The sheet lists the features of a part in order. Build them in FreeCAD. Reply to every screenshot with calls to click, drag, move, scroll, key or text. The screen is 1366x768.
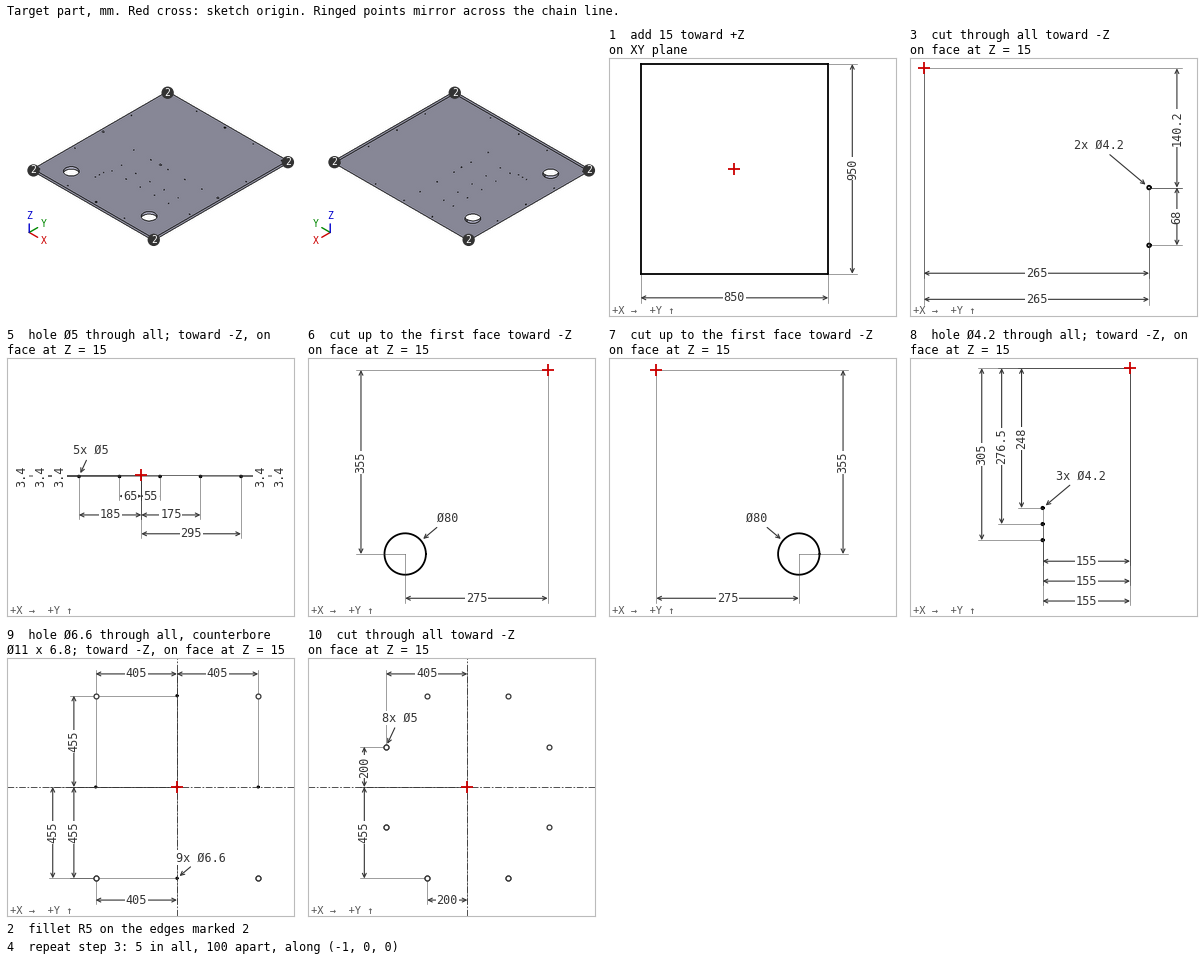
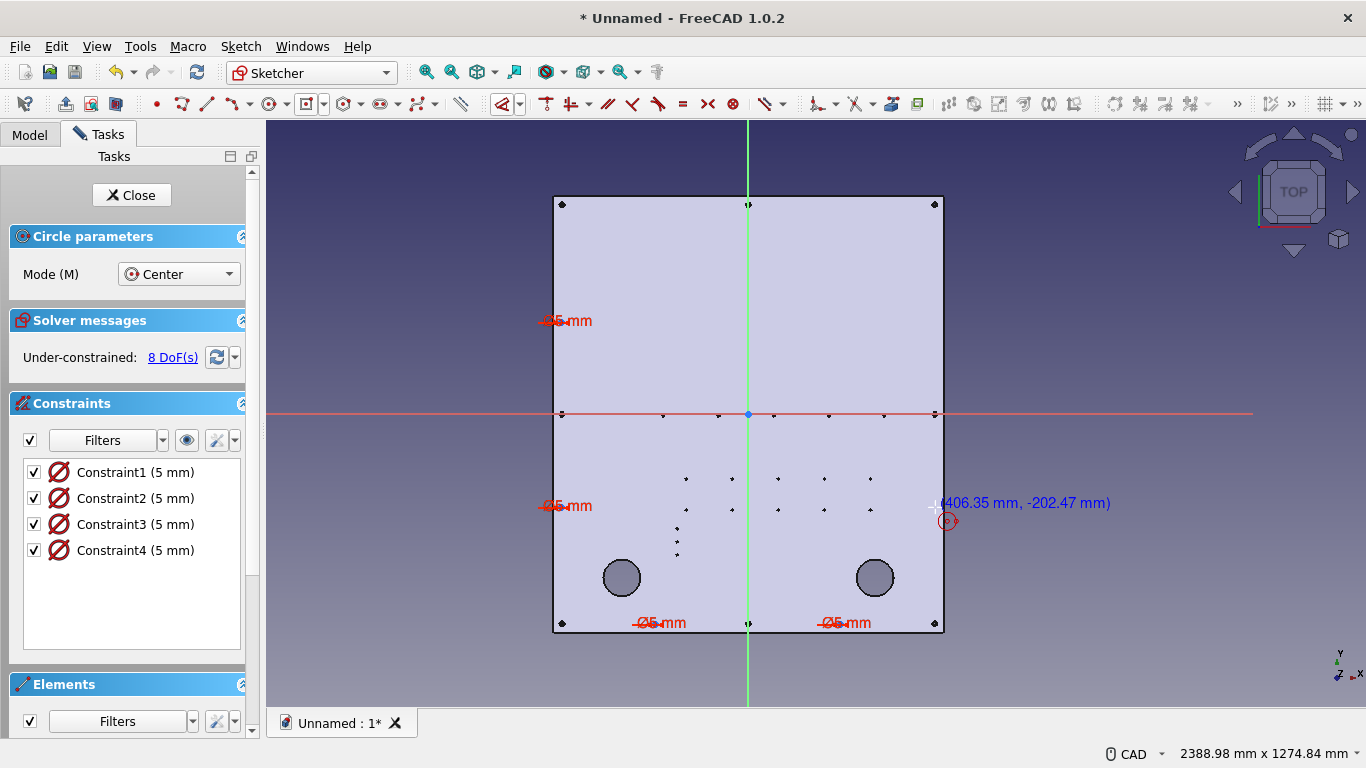
click(935, 507)
move(936, 506)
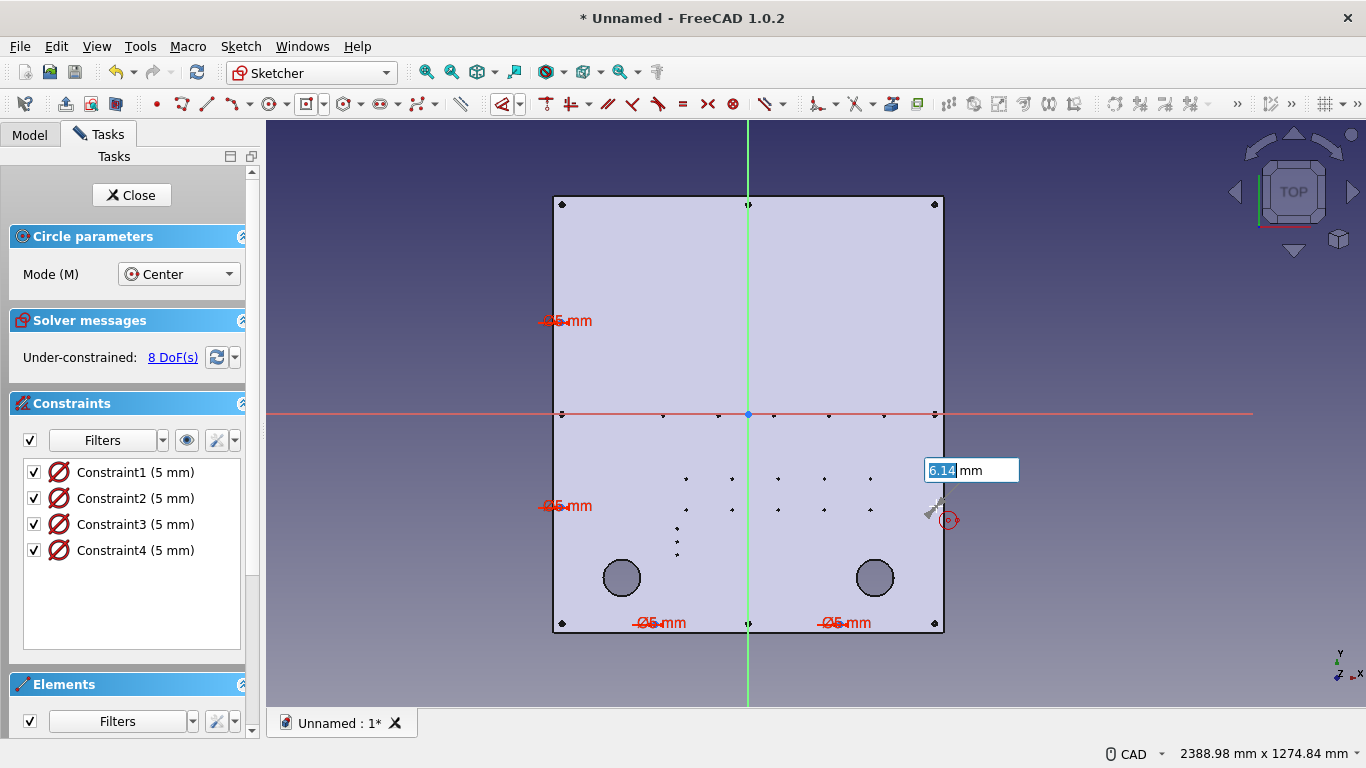
text(5)
key(Return)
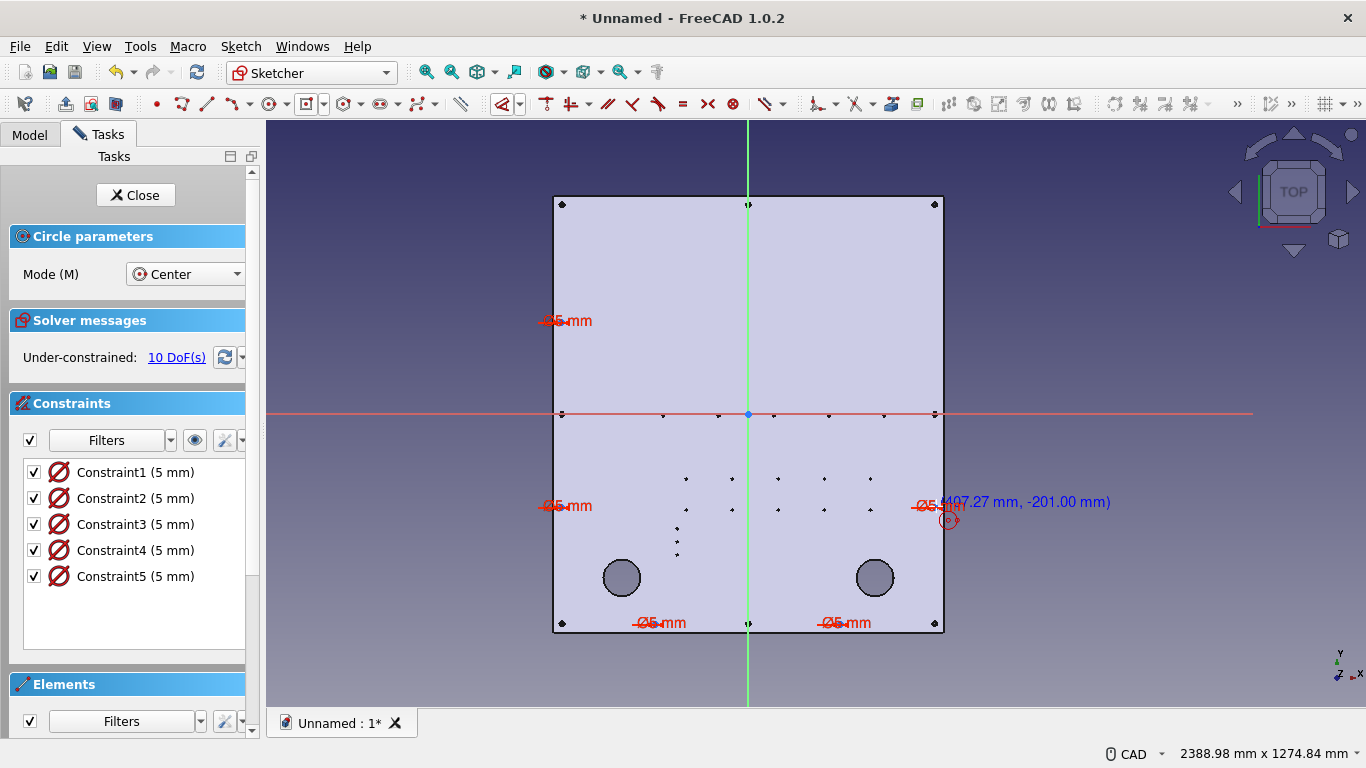
scroll(935, 322, up, 15)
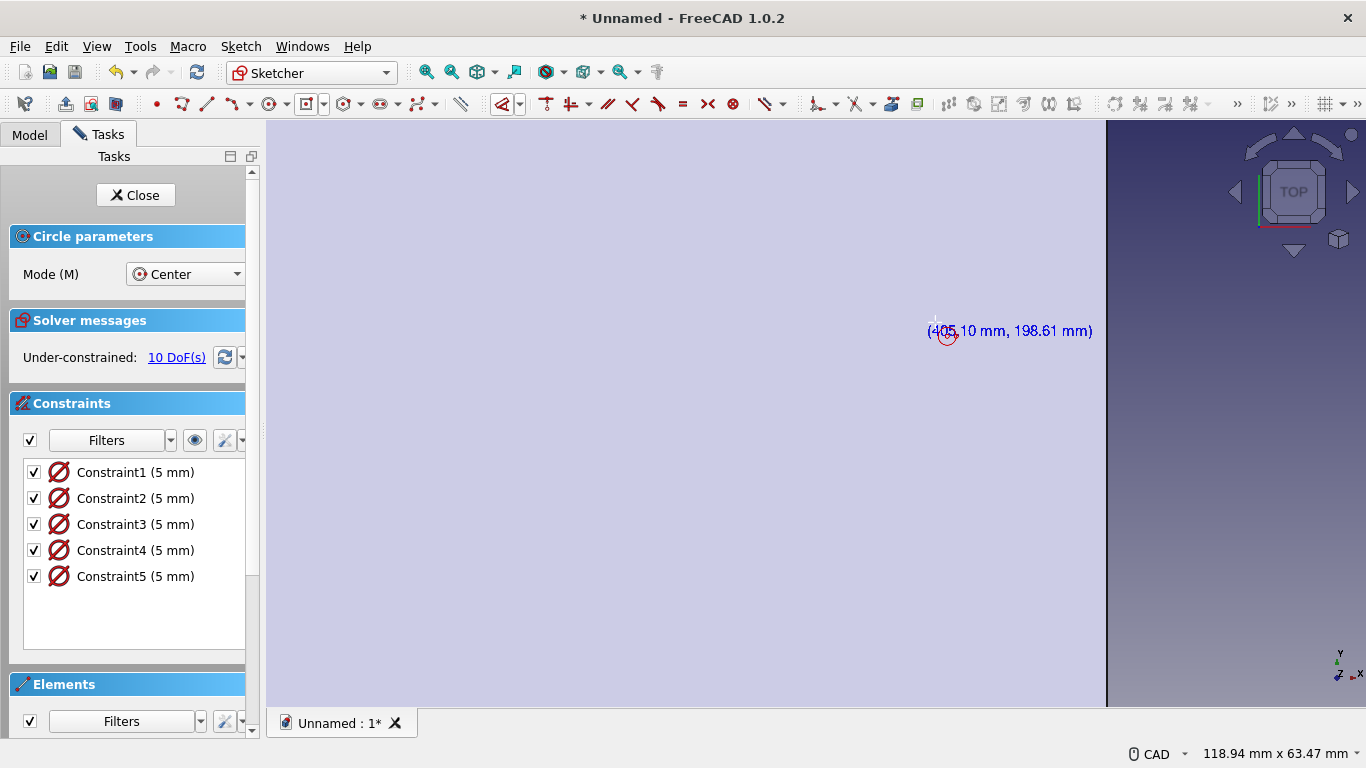
scroll(935, 321, down, 15)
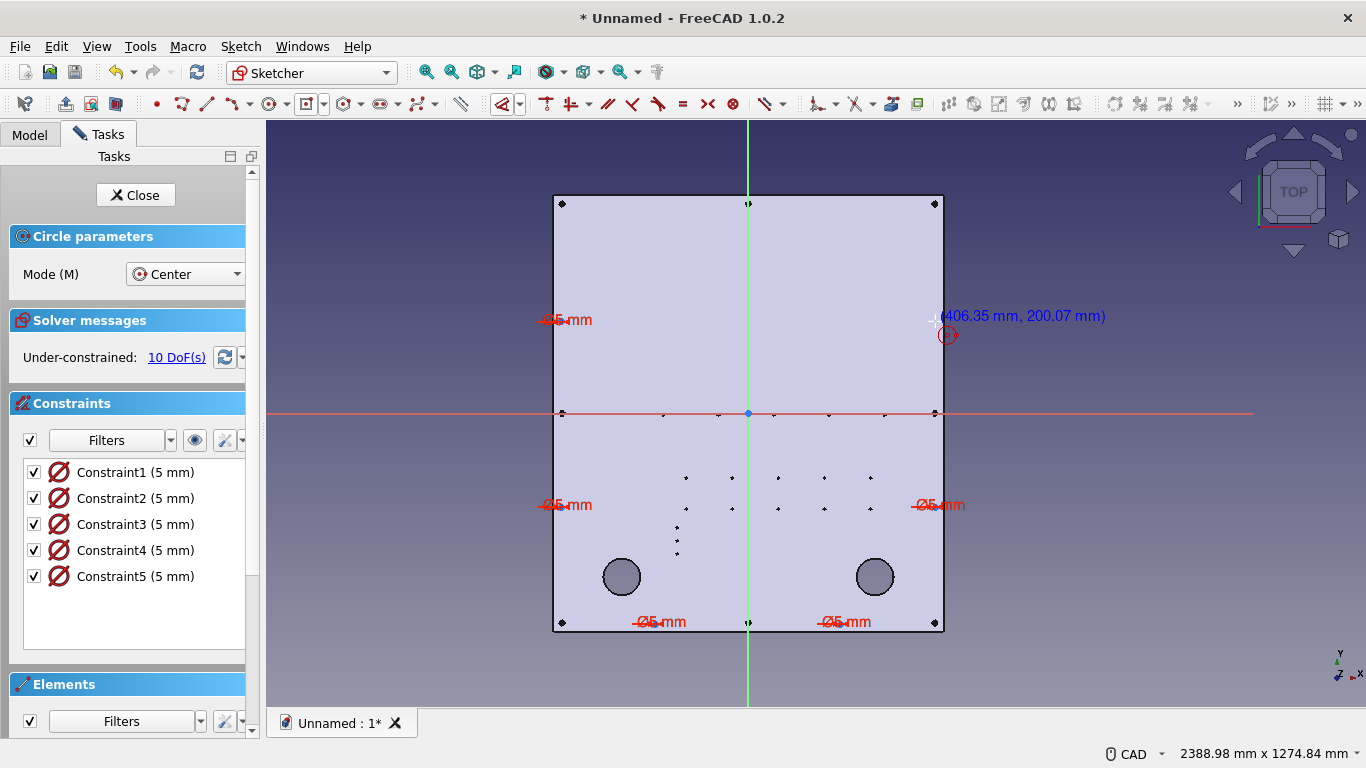
click(935, 321)
move(936, 321)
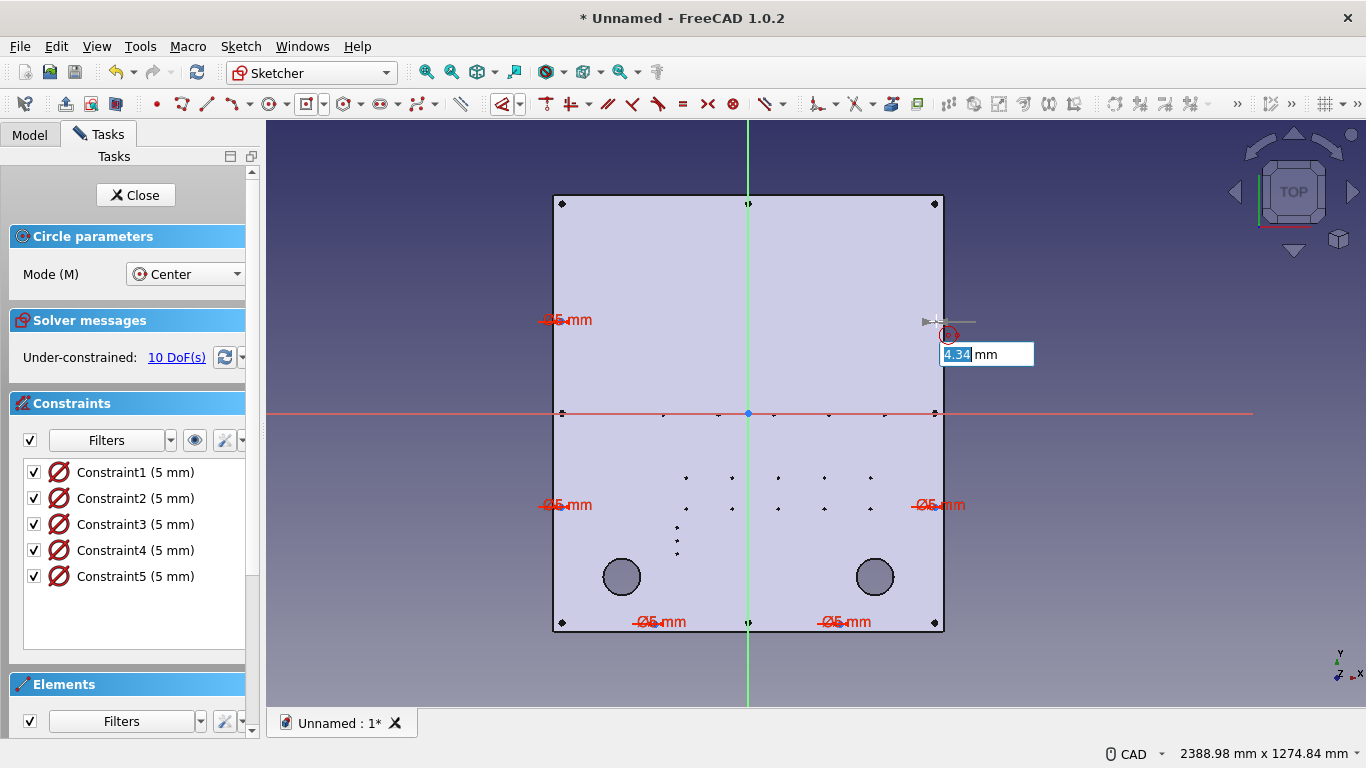
text(5)
key(Return)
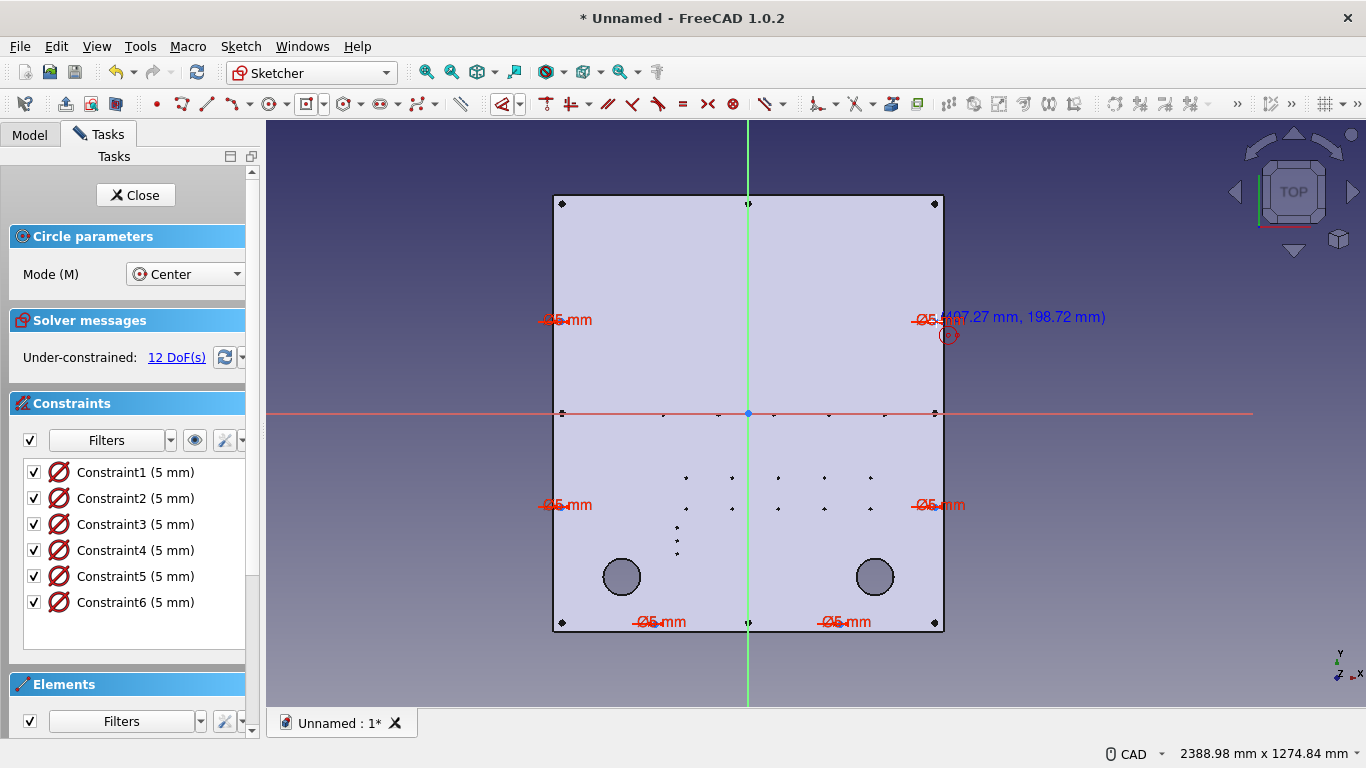
scroll(841, 204, up, 15)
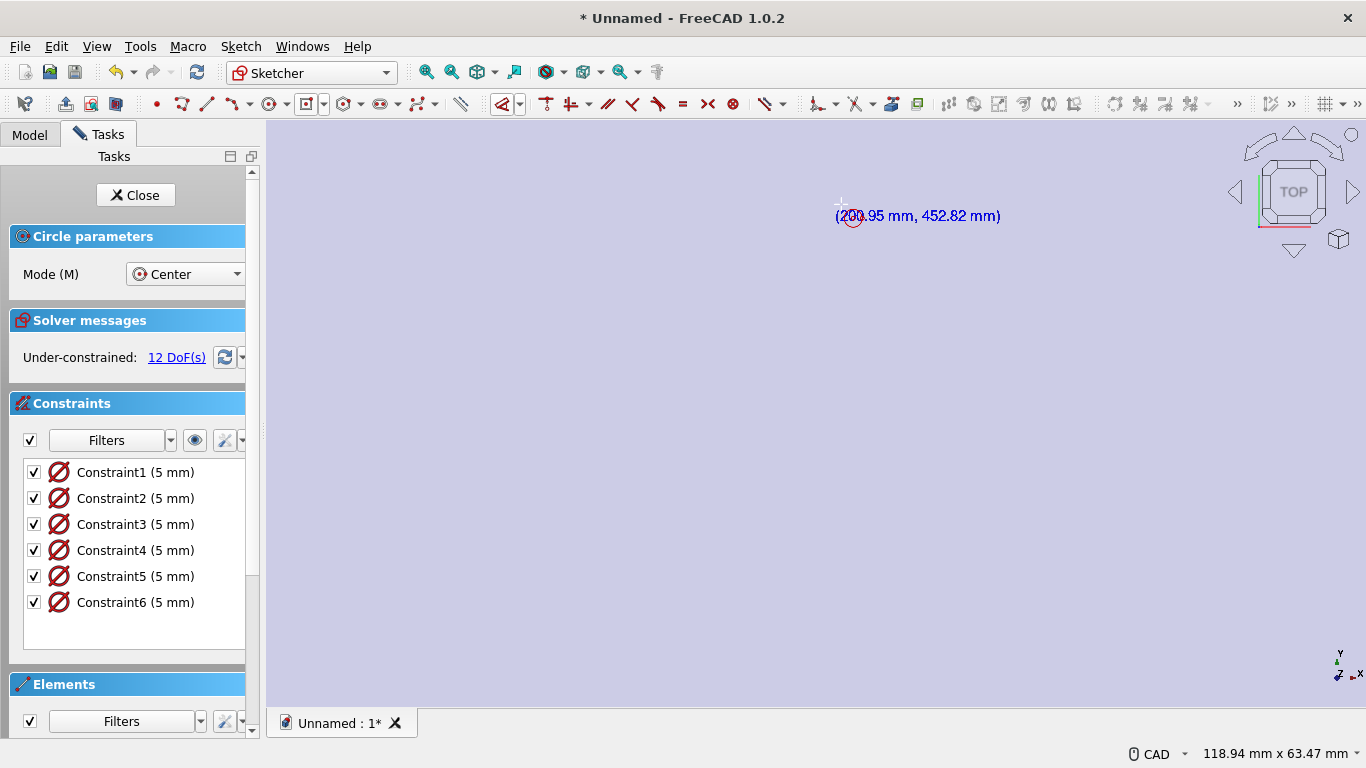
scroll(840, 204, down, 15)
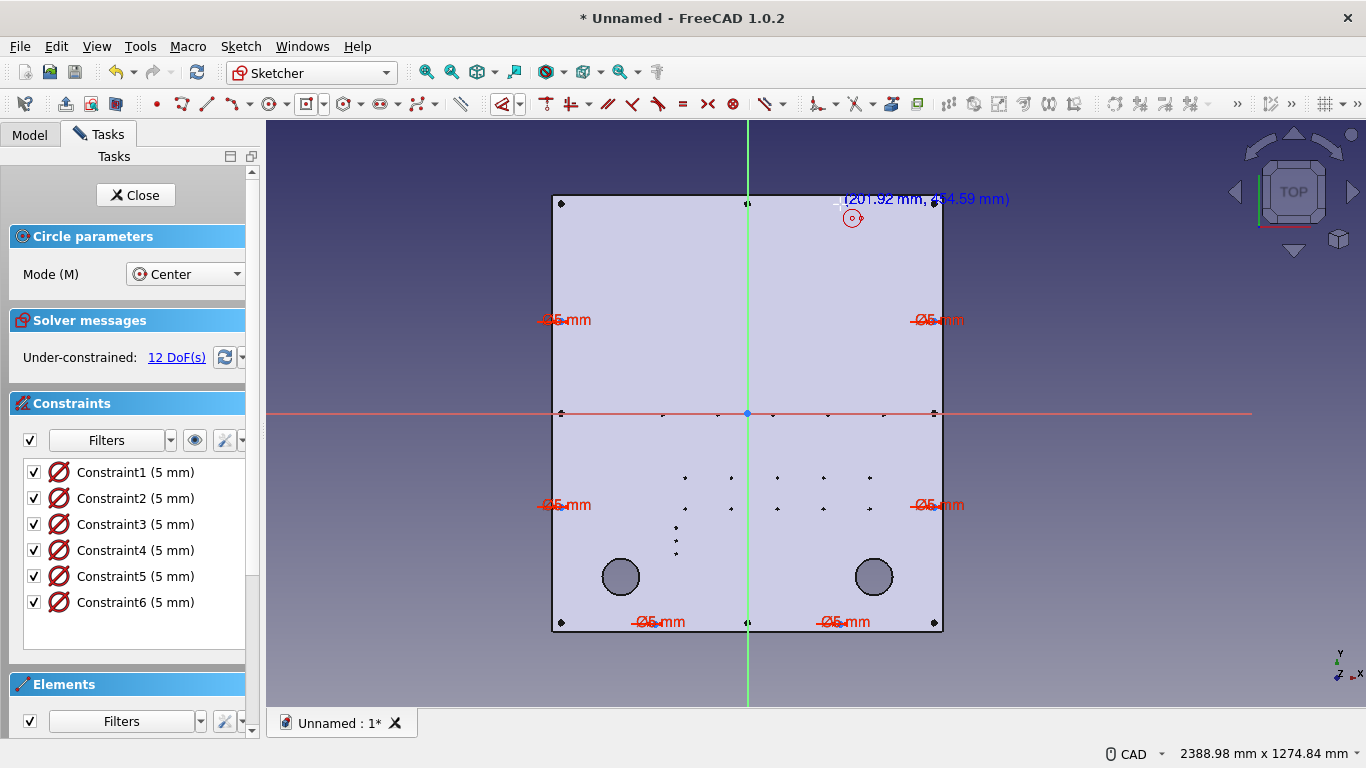
click(840, 204)
move(840, 203)